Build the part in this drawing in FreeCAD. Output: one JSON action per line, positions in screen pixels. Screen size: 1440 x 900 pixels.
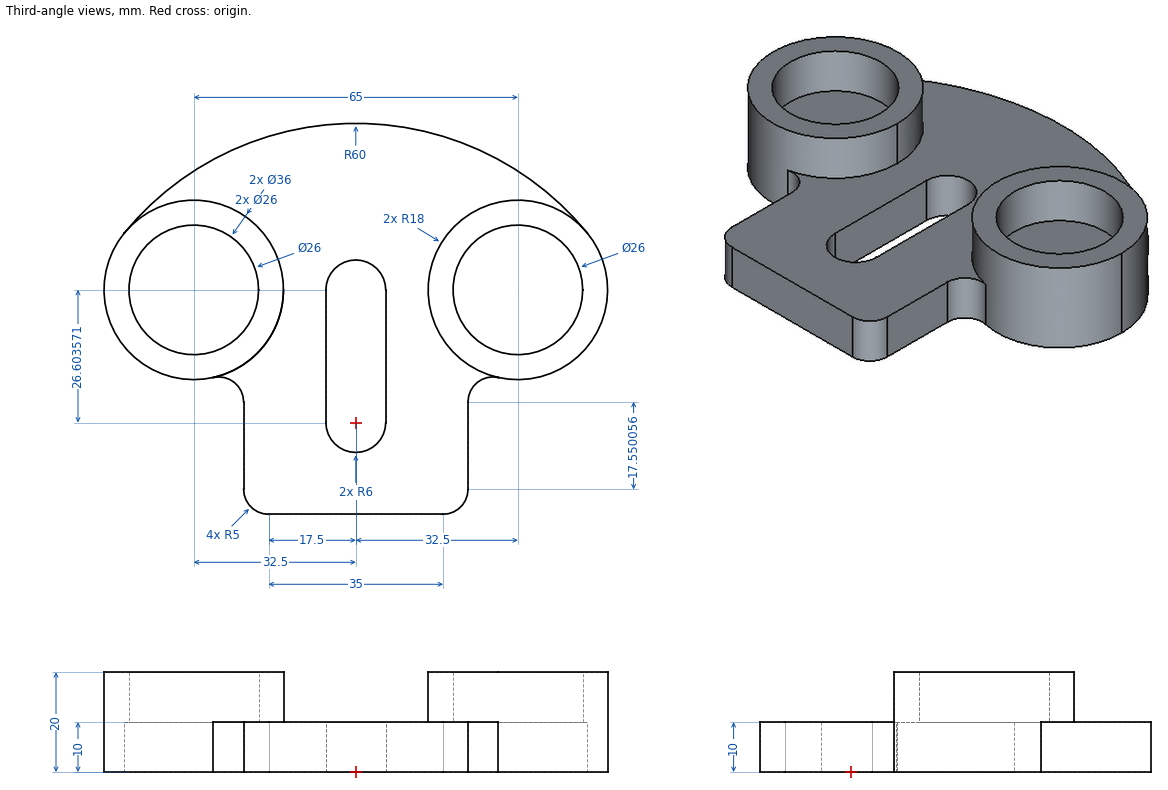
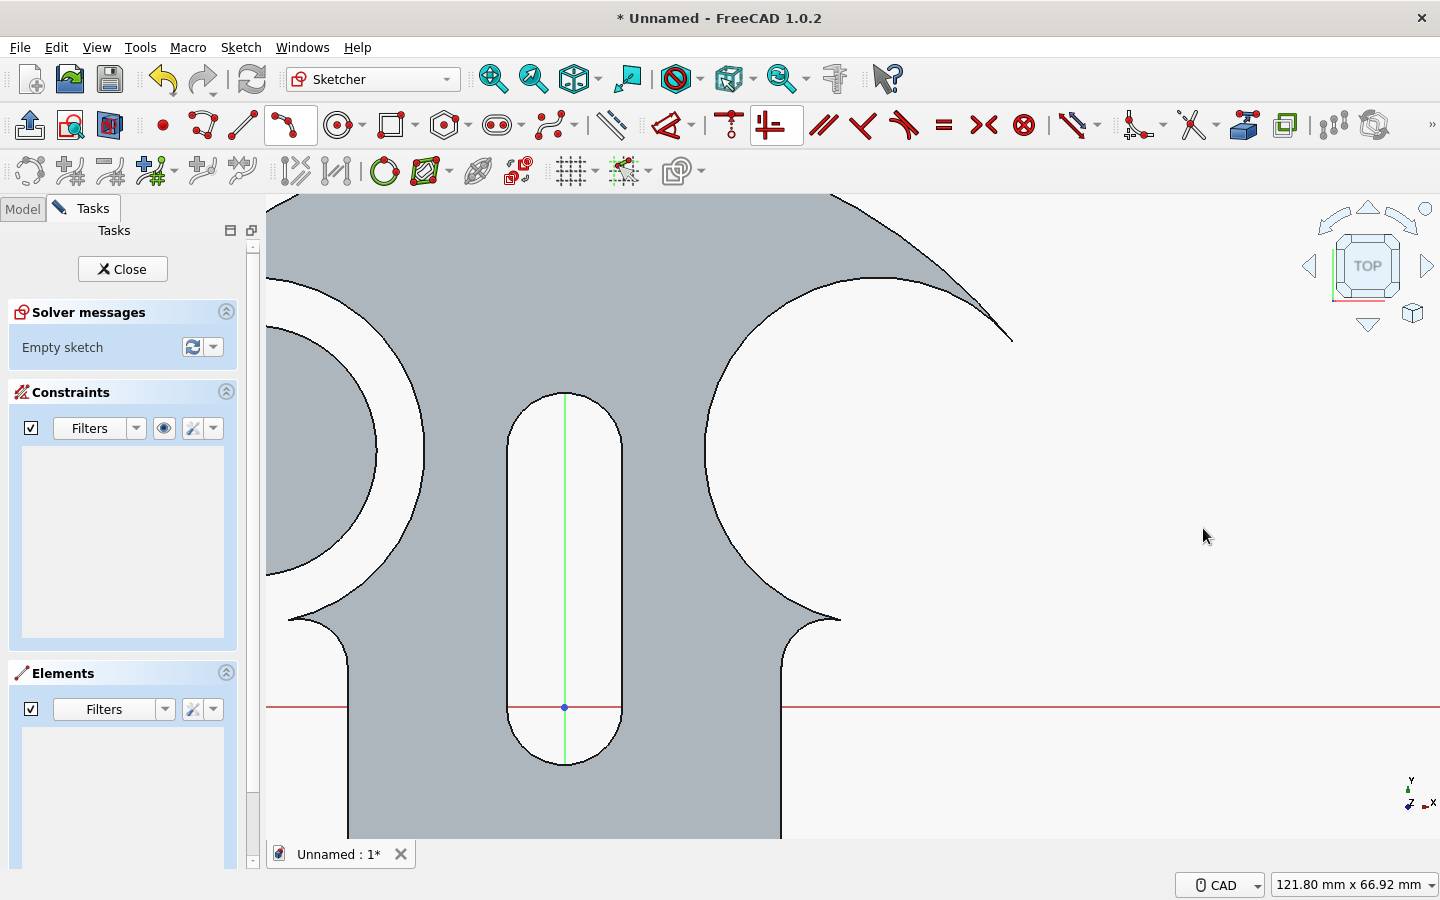
{"action": "left_click", "coordinate": [338, 126]}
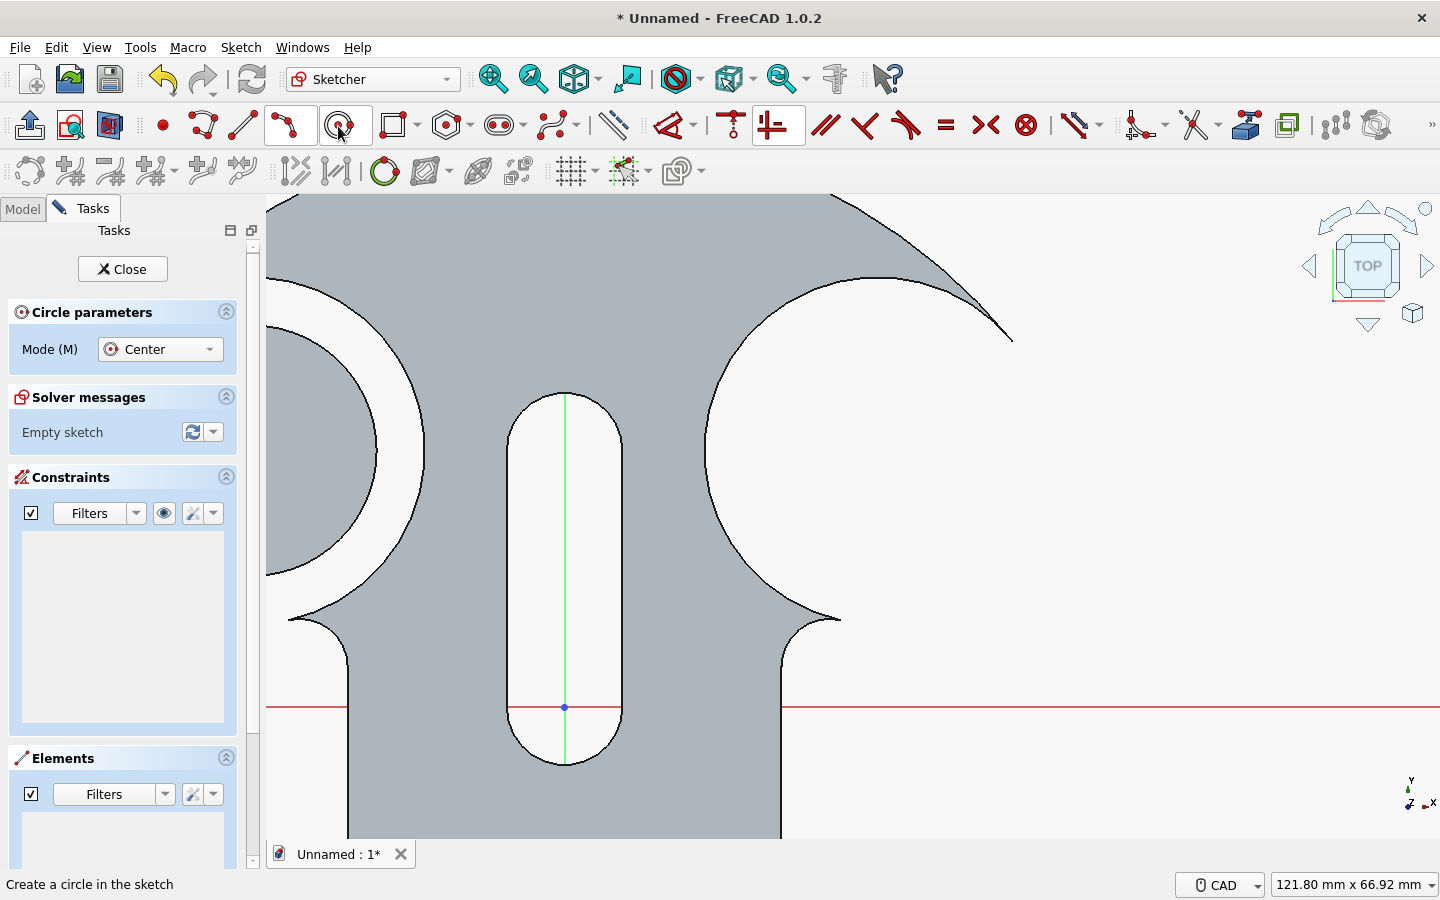
{"action": "left_click", "coordinate": [878, 451]}
{"action": "mouse_move", "coordinate": [966, 362]}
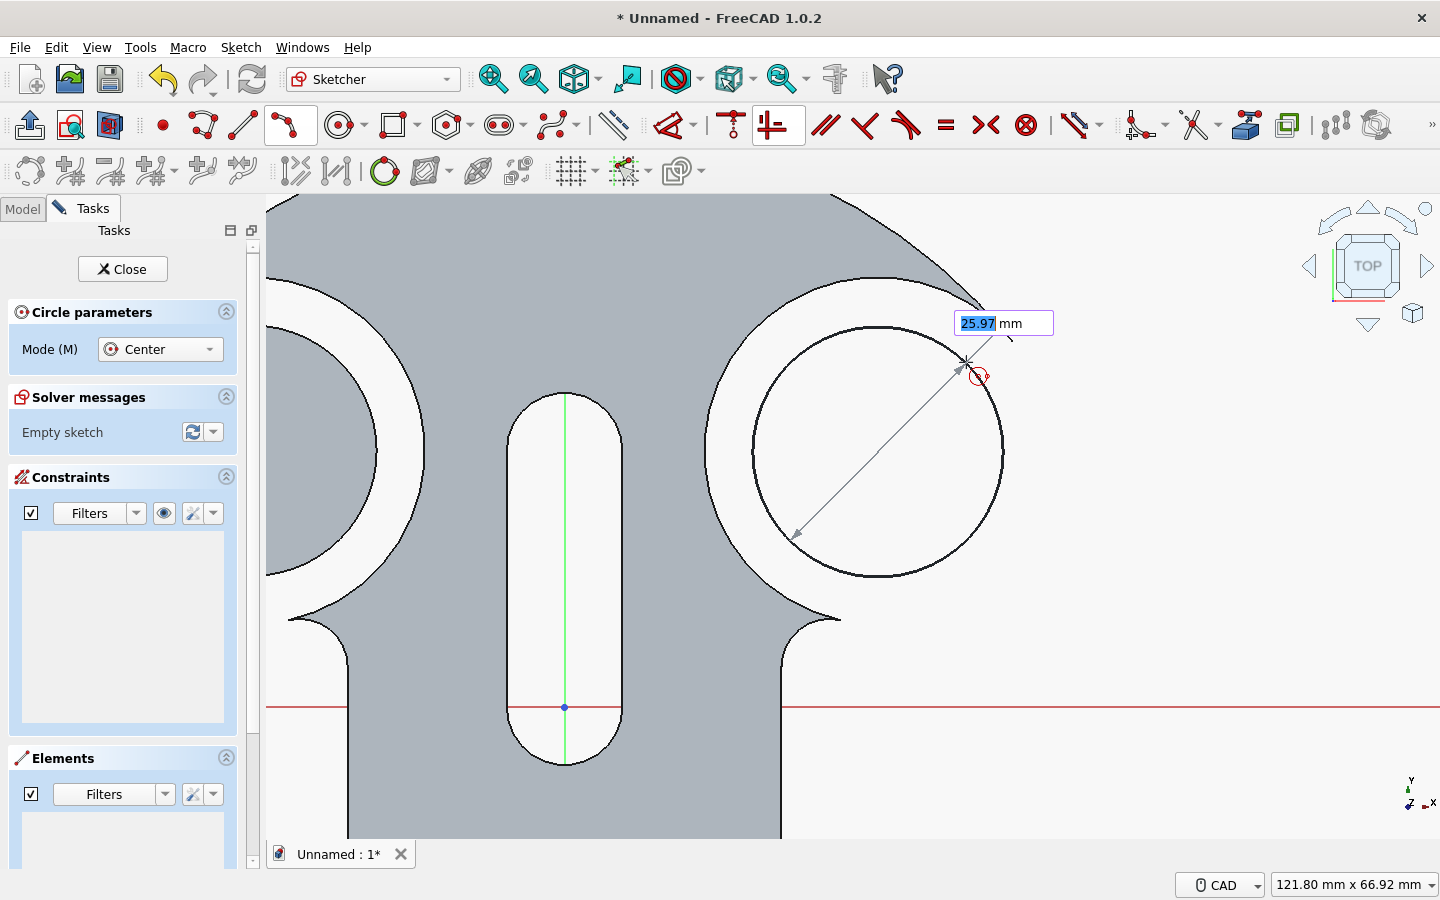
{"action": "type", "text": "26"}
{"action": "key", "text": "Return"}
{"action": "key", "text": "Escape"}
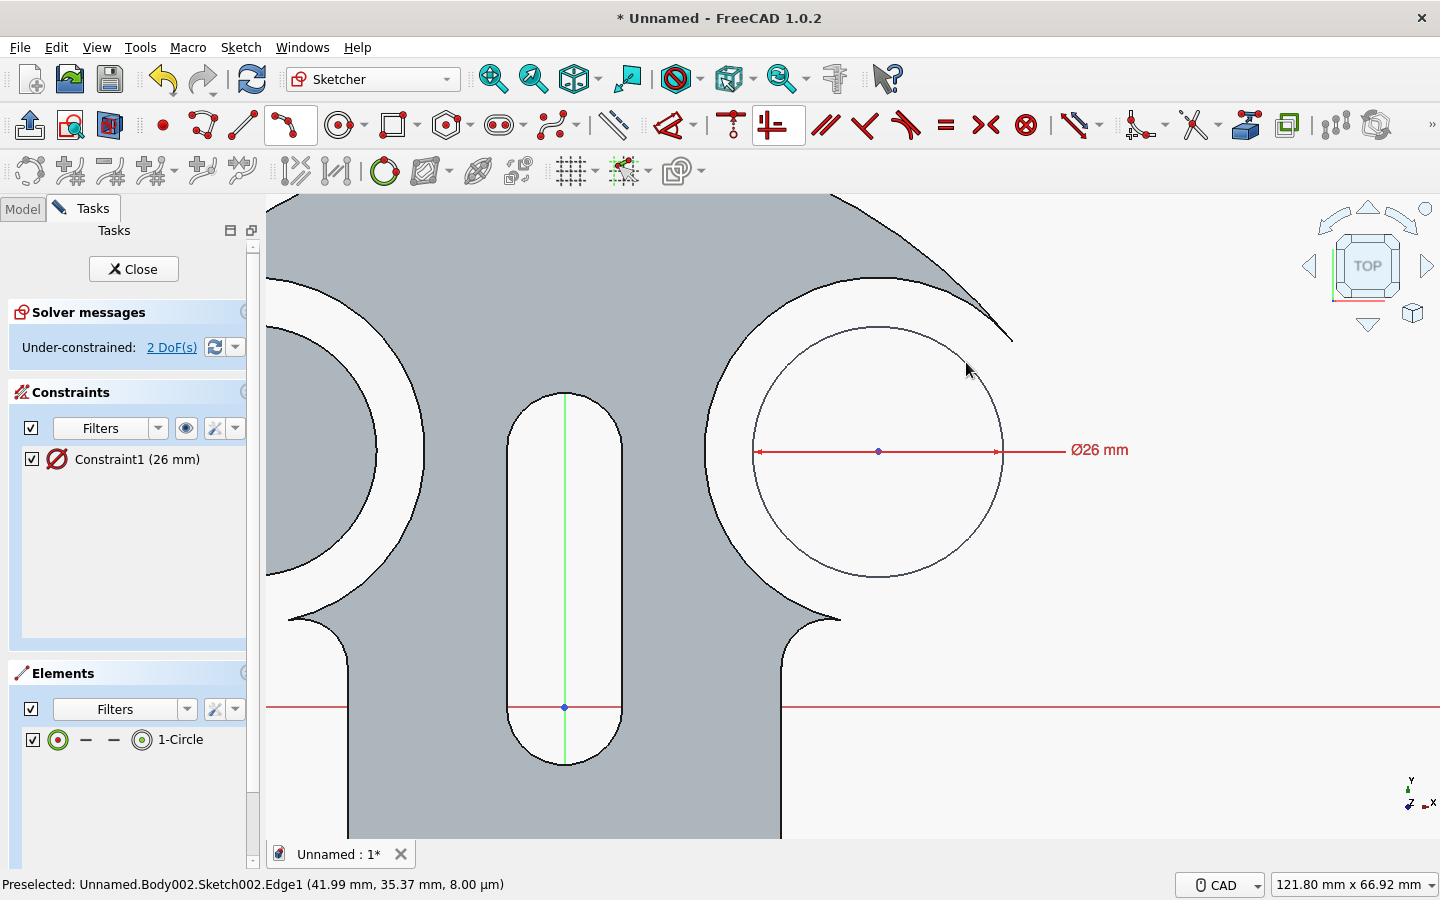
{"action": "key", "text": "d"}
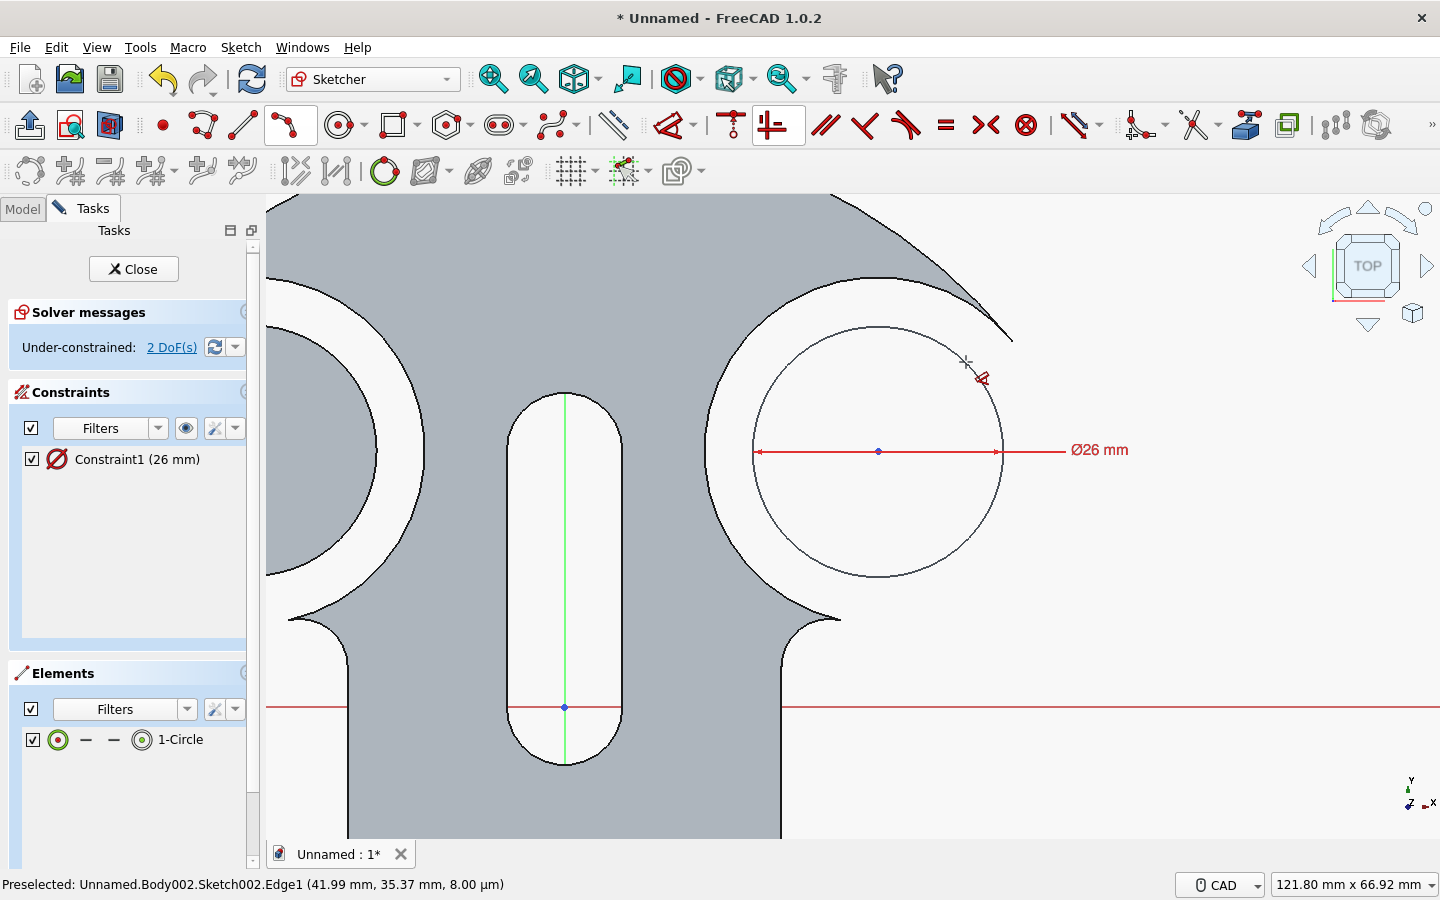
{"action": "left_click", "coordinate": [878, 452]}
{"action": "left_click", "coordinate": [721, 741]}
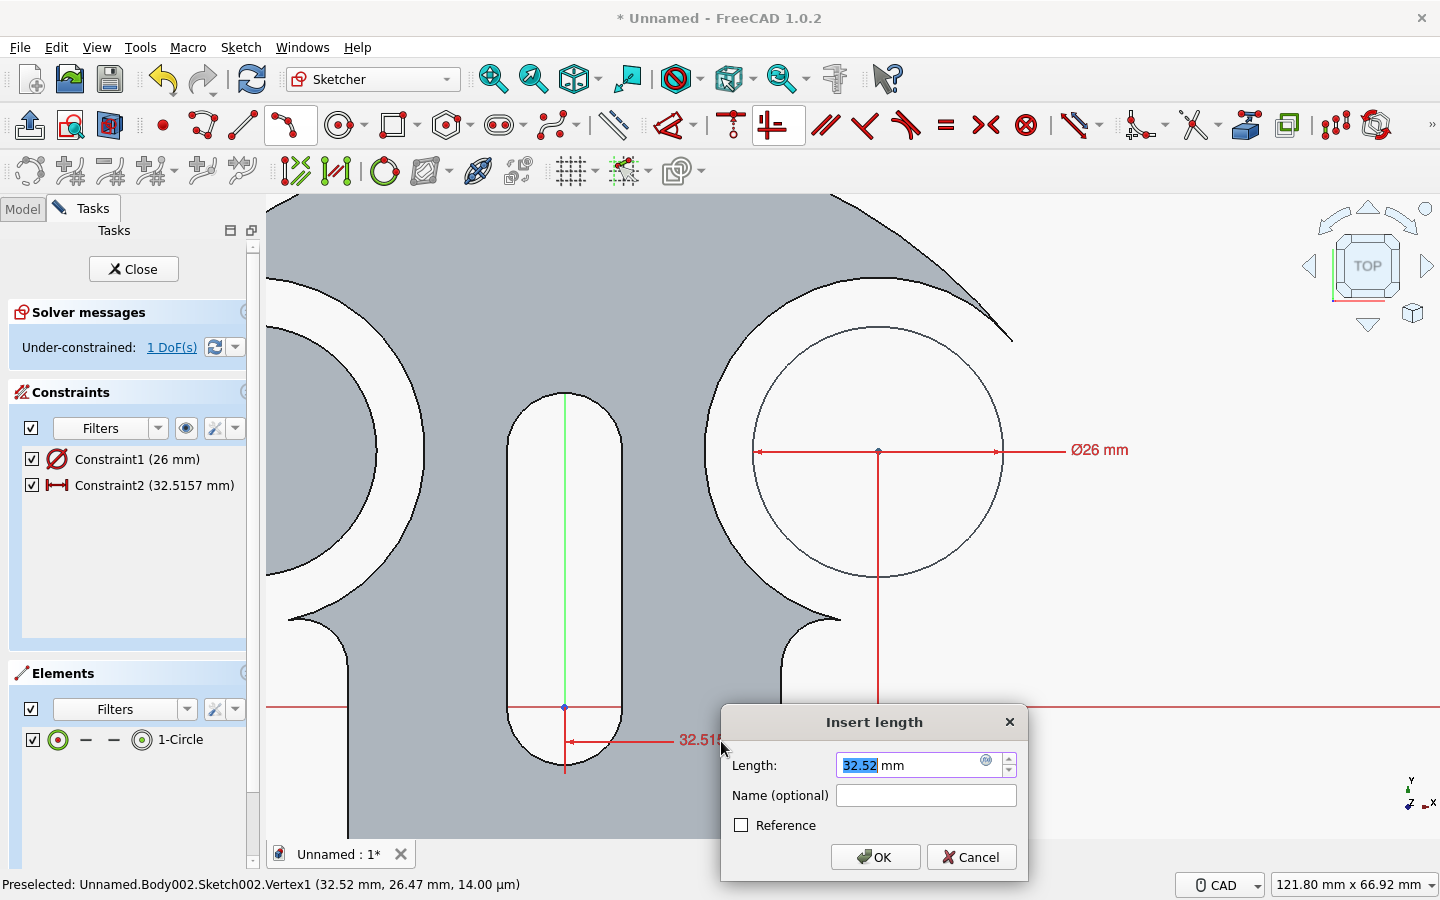
{"action": "type", "text": "32.5"}
{"action": "key", "text": "Return"}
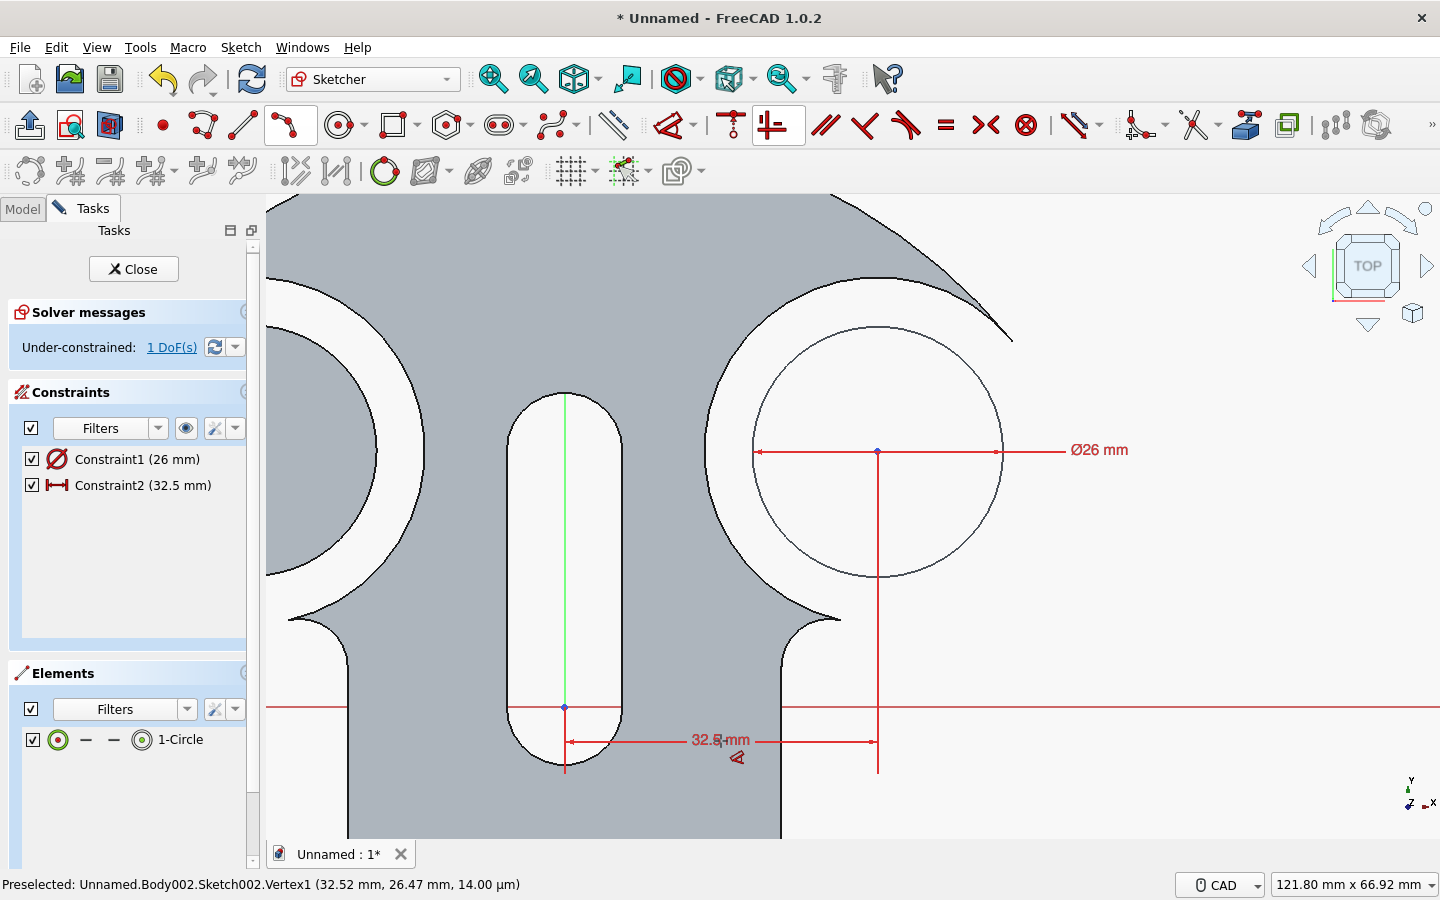
{"action": "left_click", "coordinate": [878, 452]}
{"action": "left_click", "coordinate": [531, 580]}